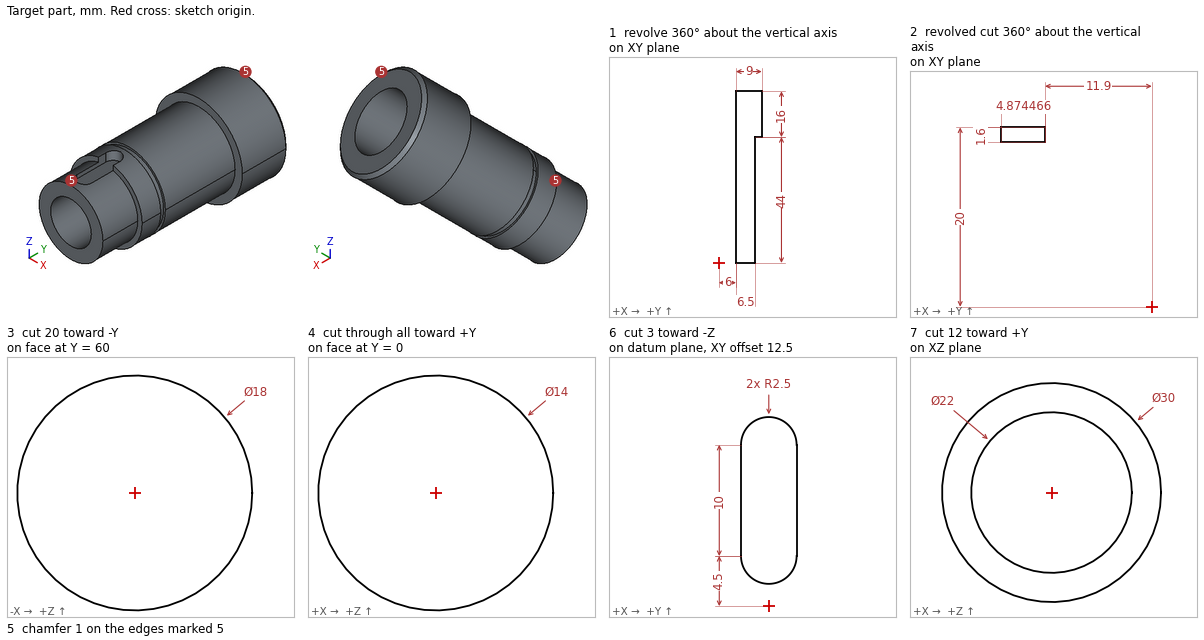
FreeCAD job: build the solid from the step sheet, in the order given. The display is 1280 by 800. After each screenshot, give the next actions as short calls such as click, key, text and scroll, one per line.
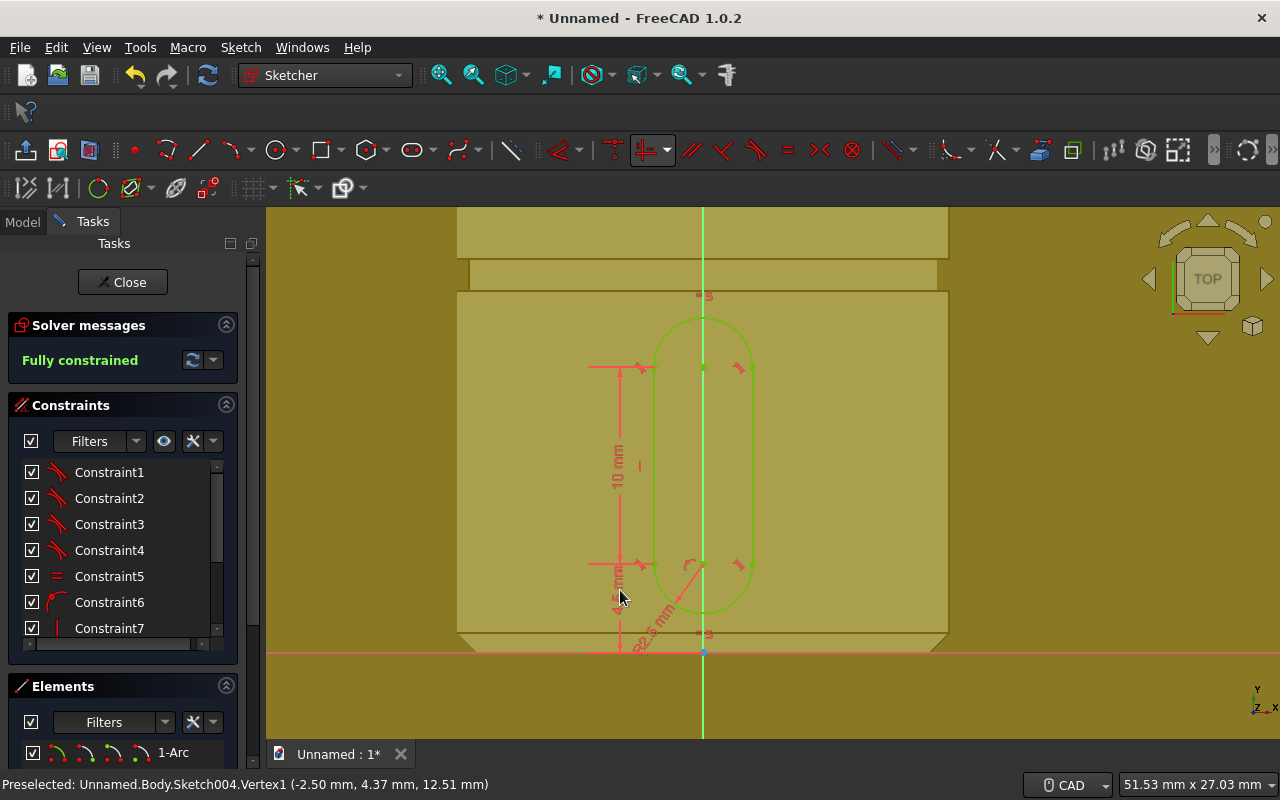
click(123, 282)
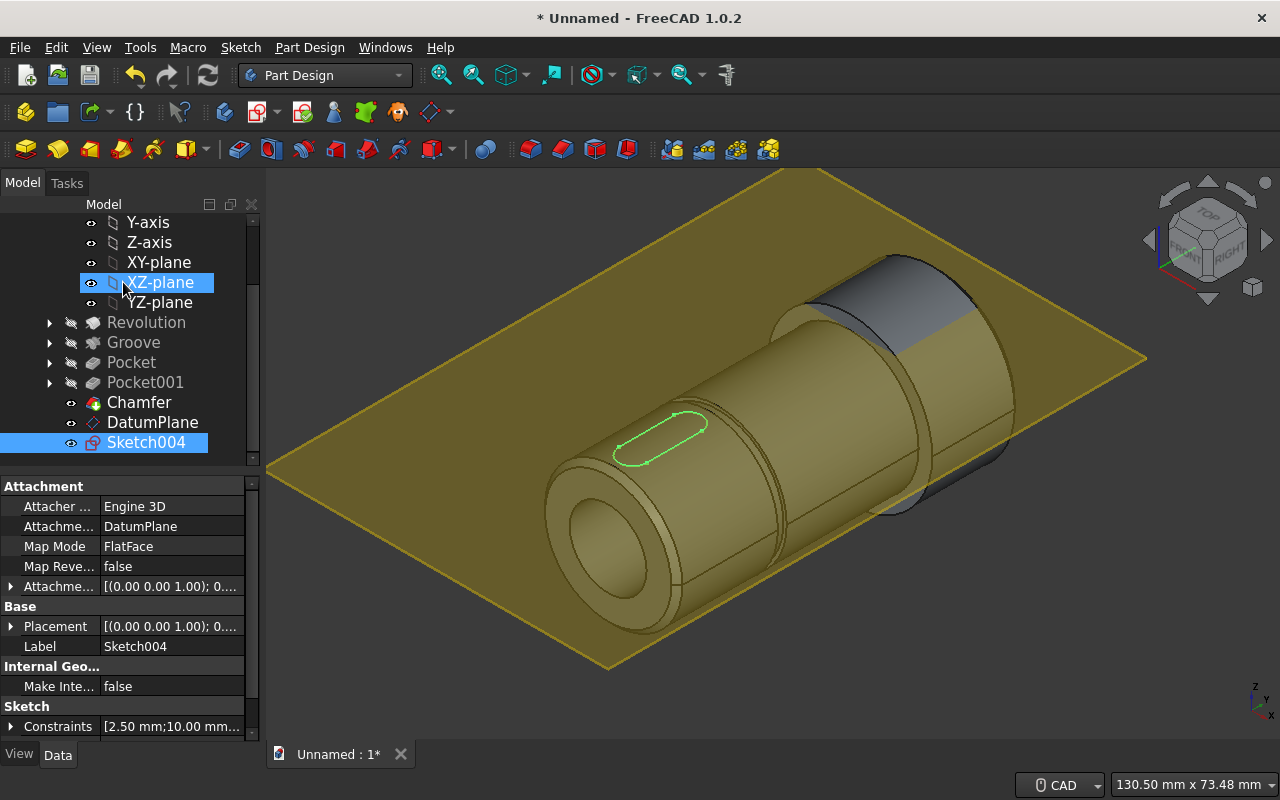
click(240, 150)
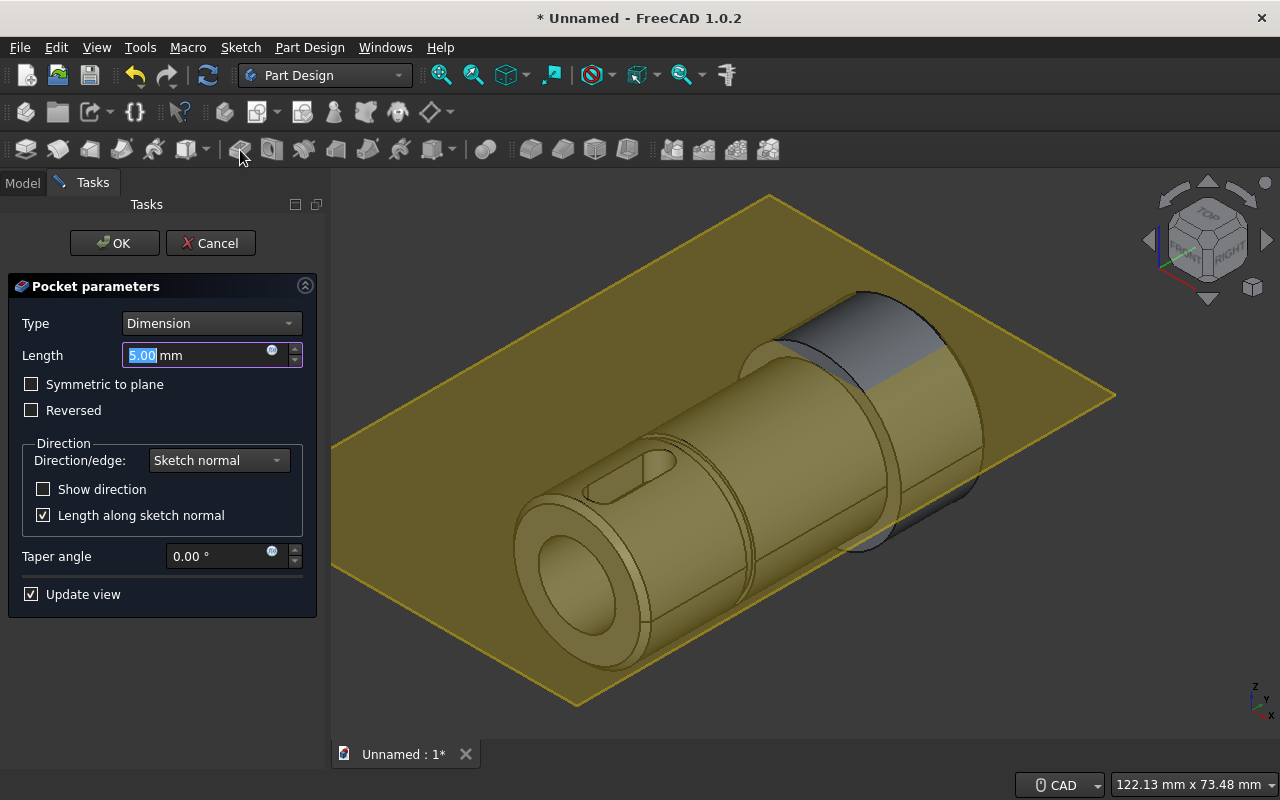
text(3)
key(Tab)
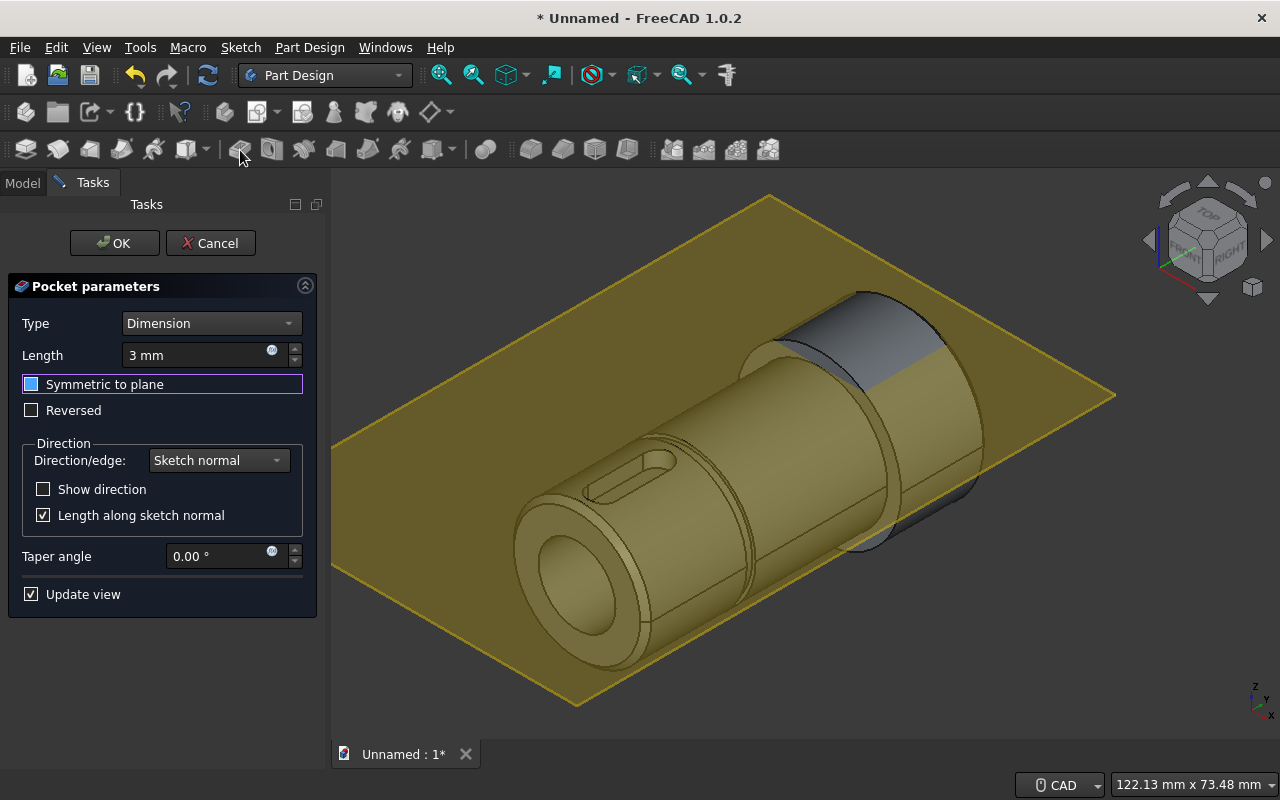
click(115, 243)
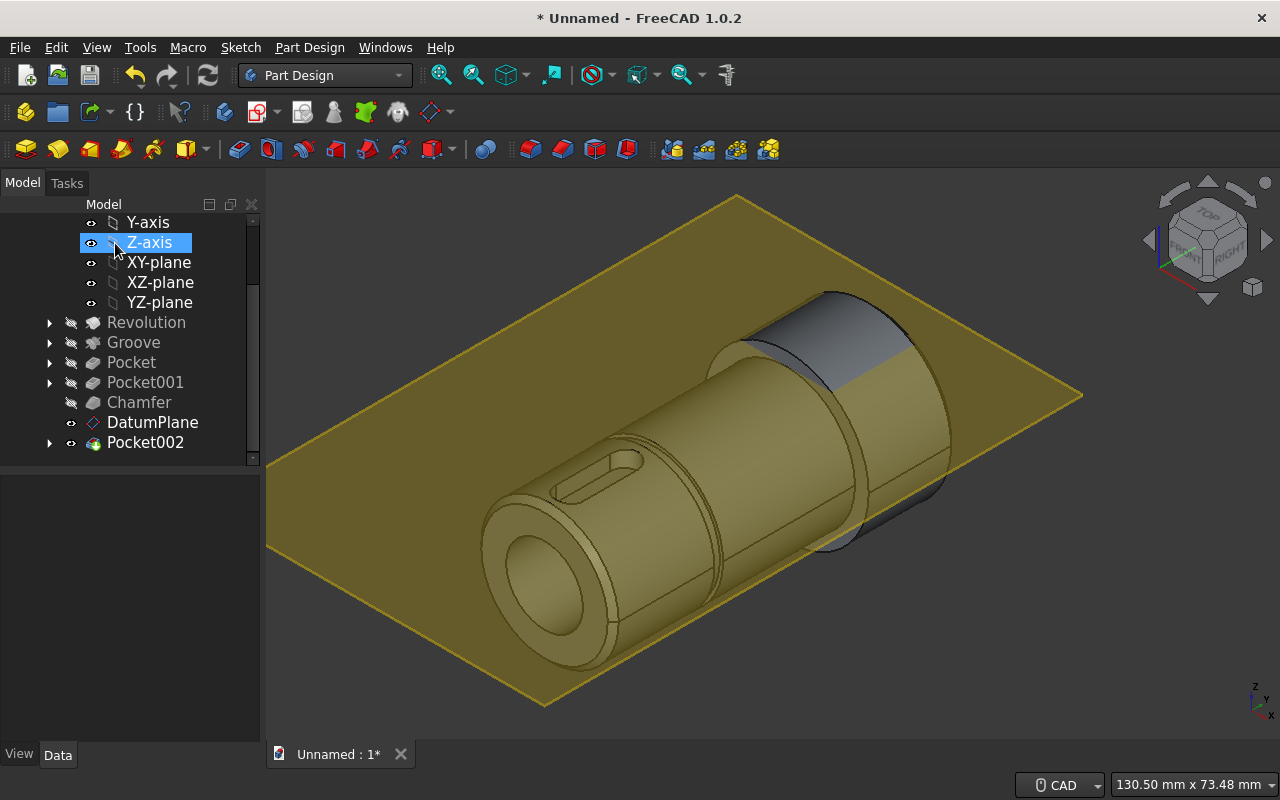
click(116, 423)
key(space)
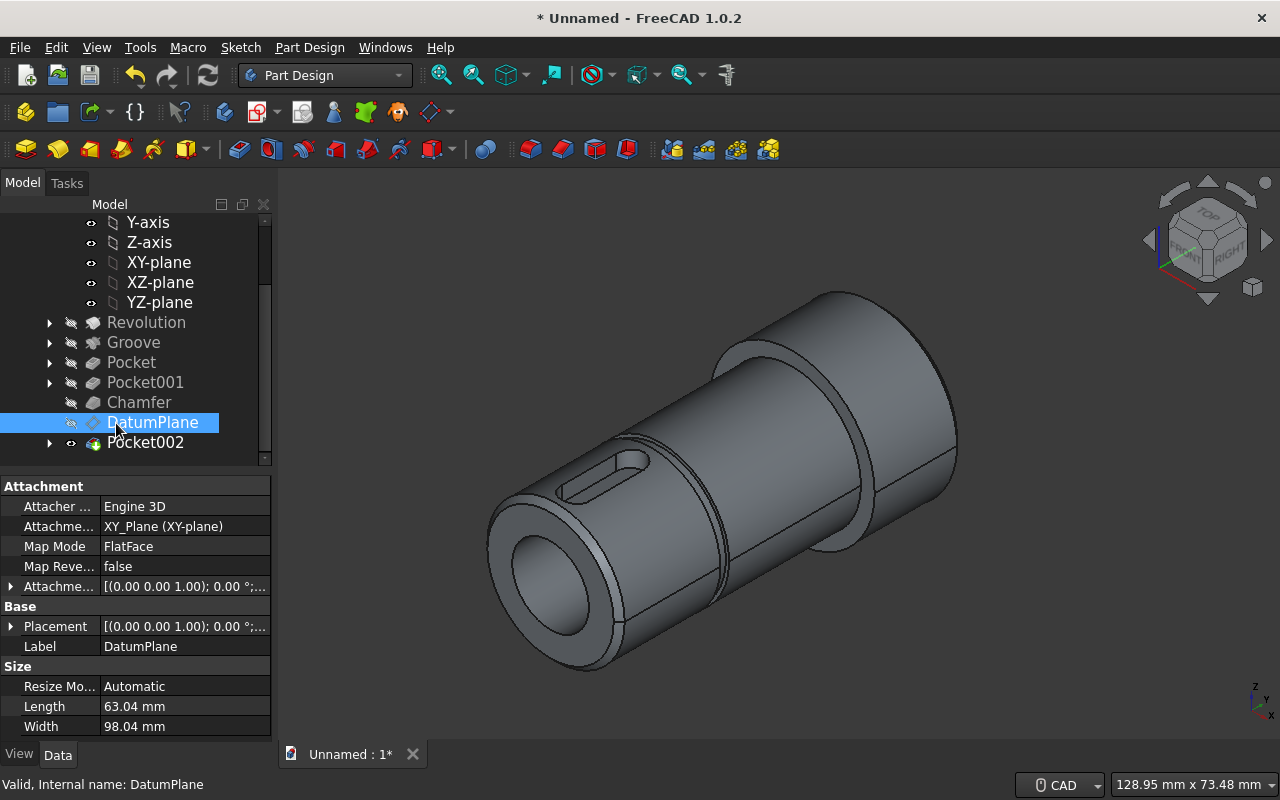
click(318, 699)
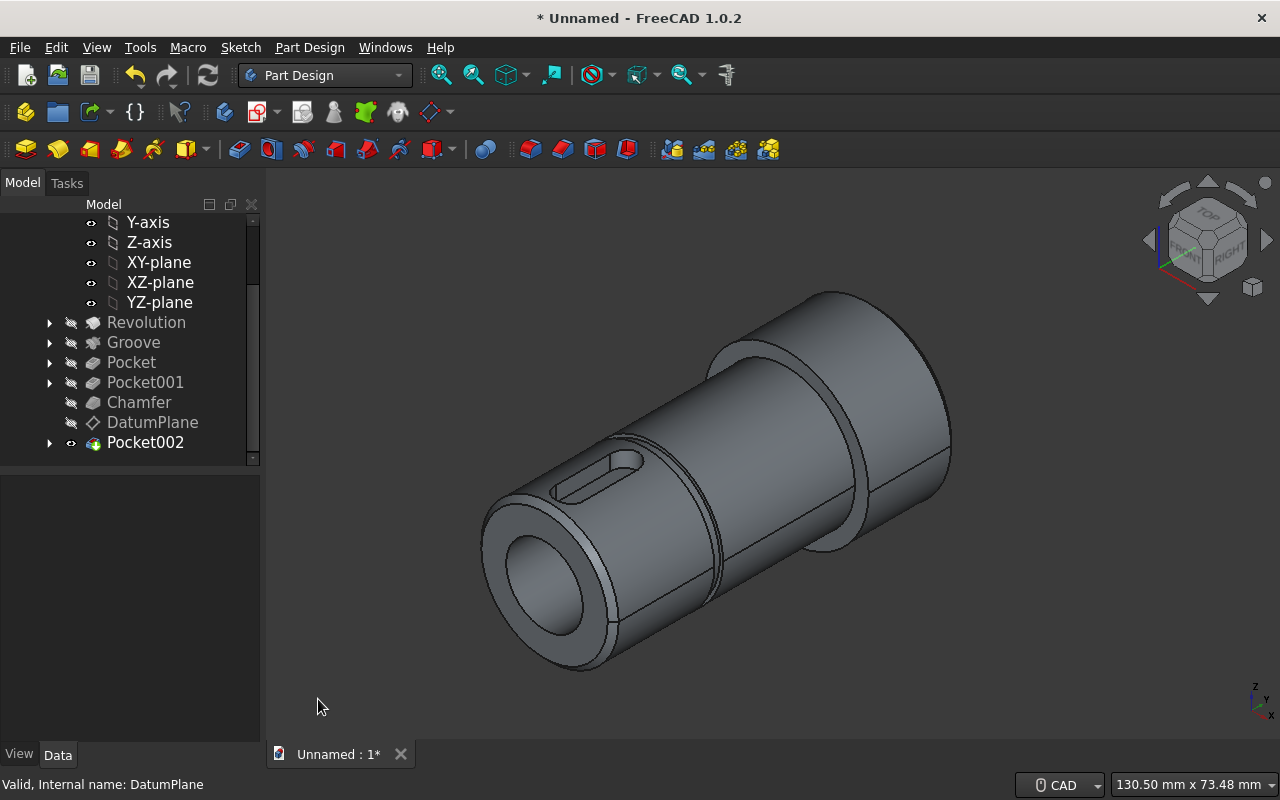
click(258, 112)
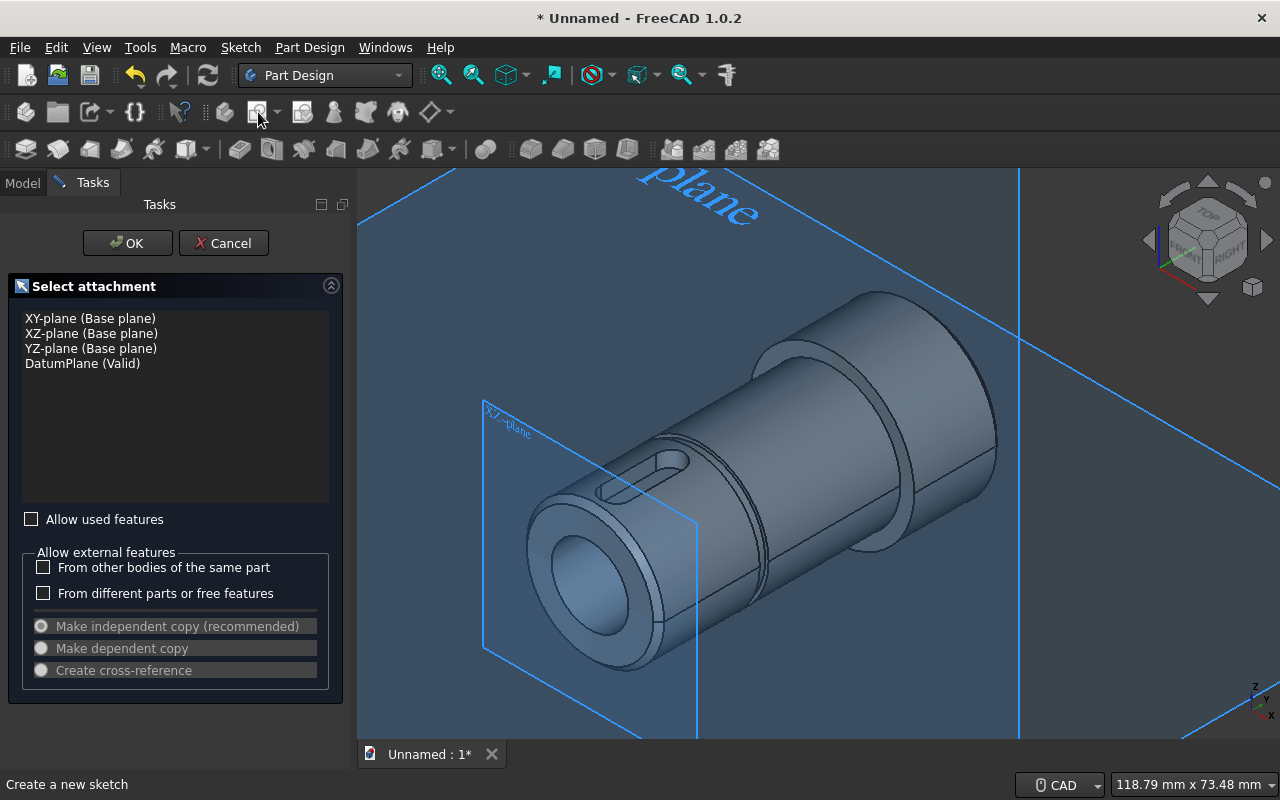
click(82, 334)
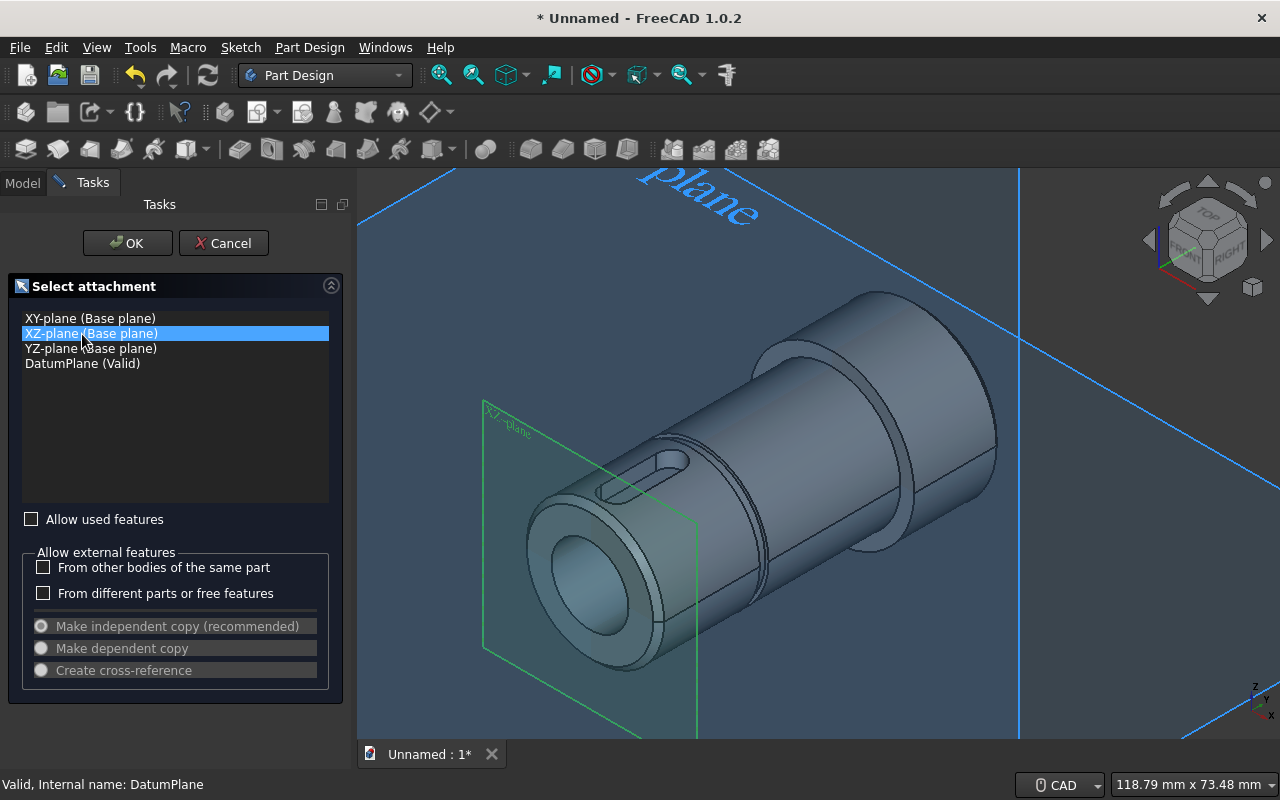
click(128, 243)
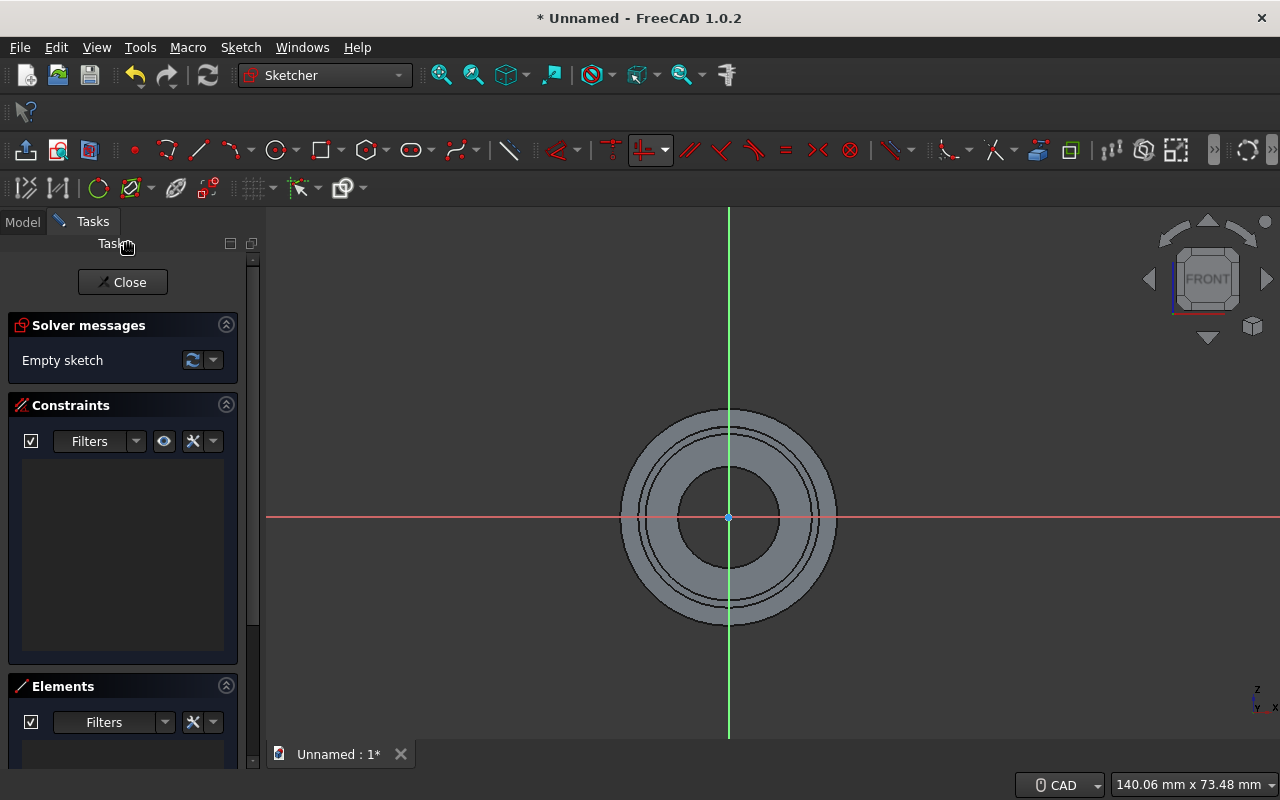
scroll(778, 607, up, 2)